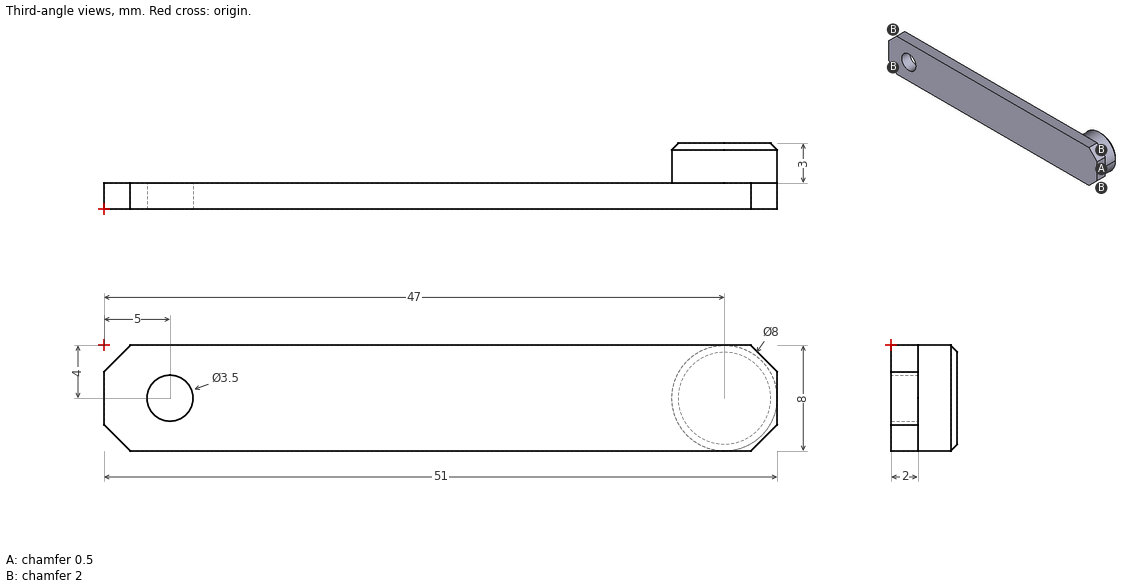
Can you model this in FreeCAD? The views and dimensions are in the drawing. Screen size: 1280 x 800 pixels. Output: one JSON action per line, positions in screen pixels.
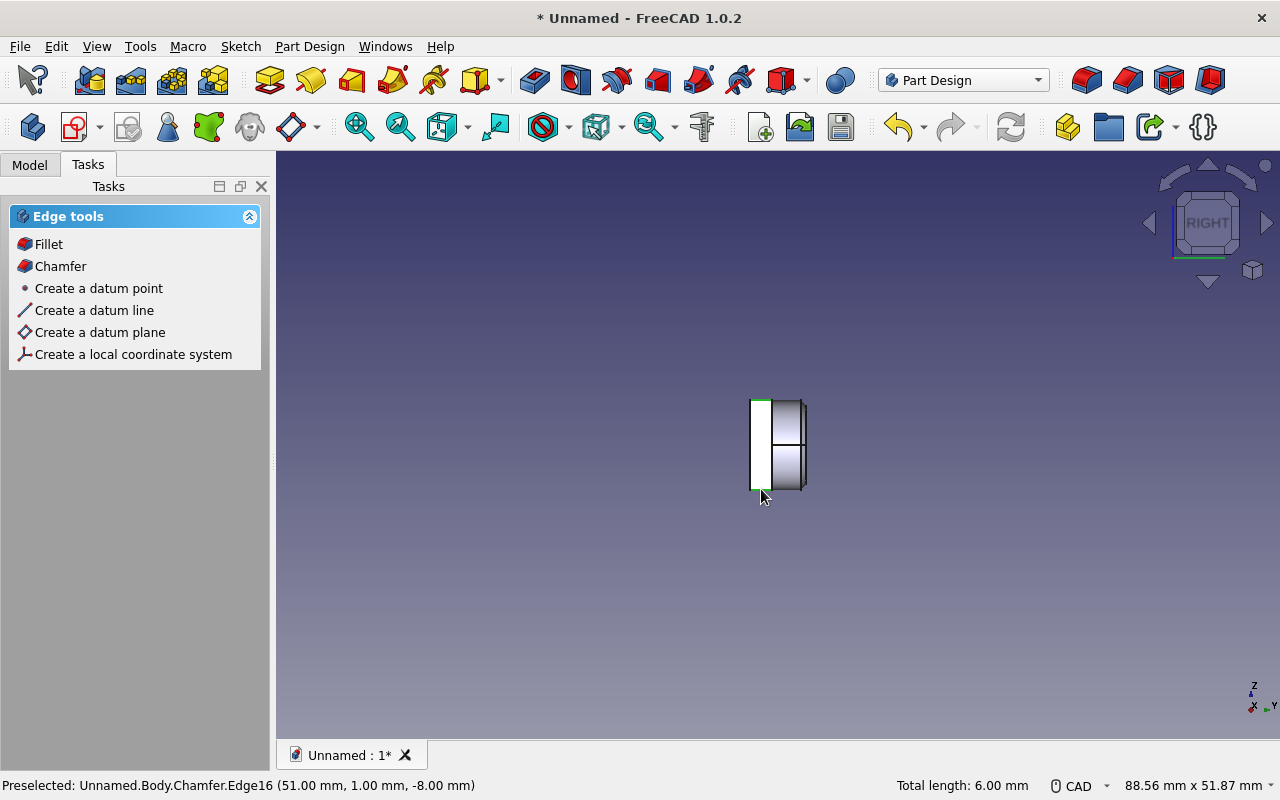
{"action": "key", "text": "5"}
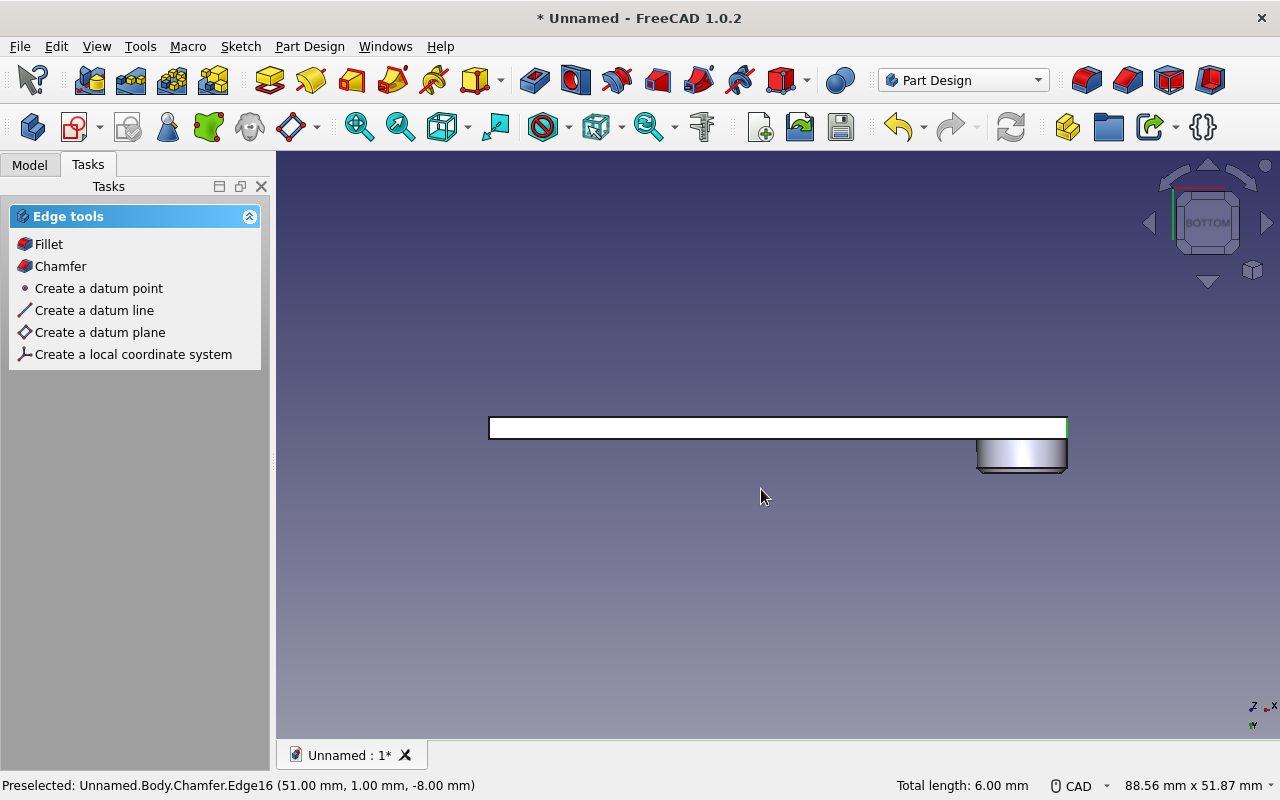
{"action": "left_click", "coordinate": [489, 427], "text": "ctrl"}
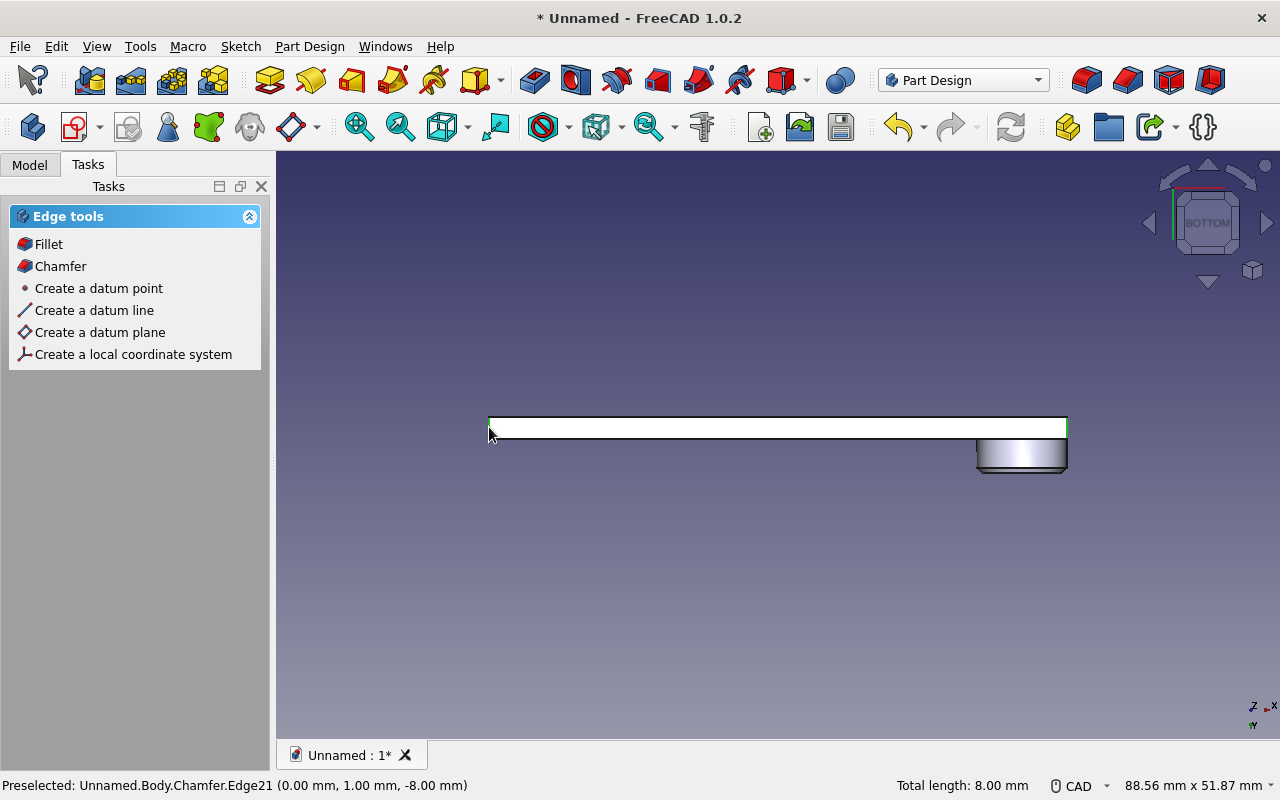
{"action": "left_click", "coordinate": [1128, 80]}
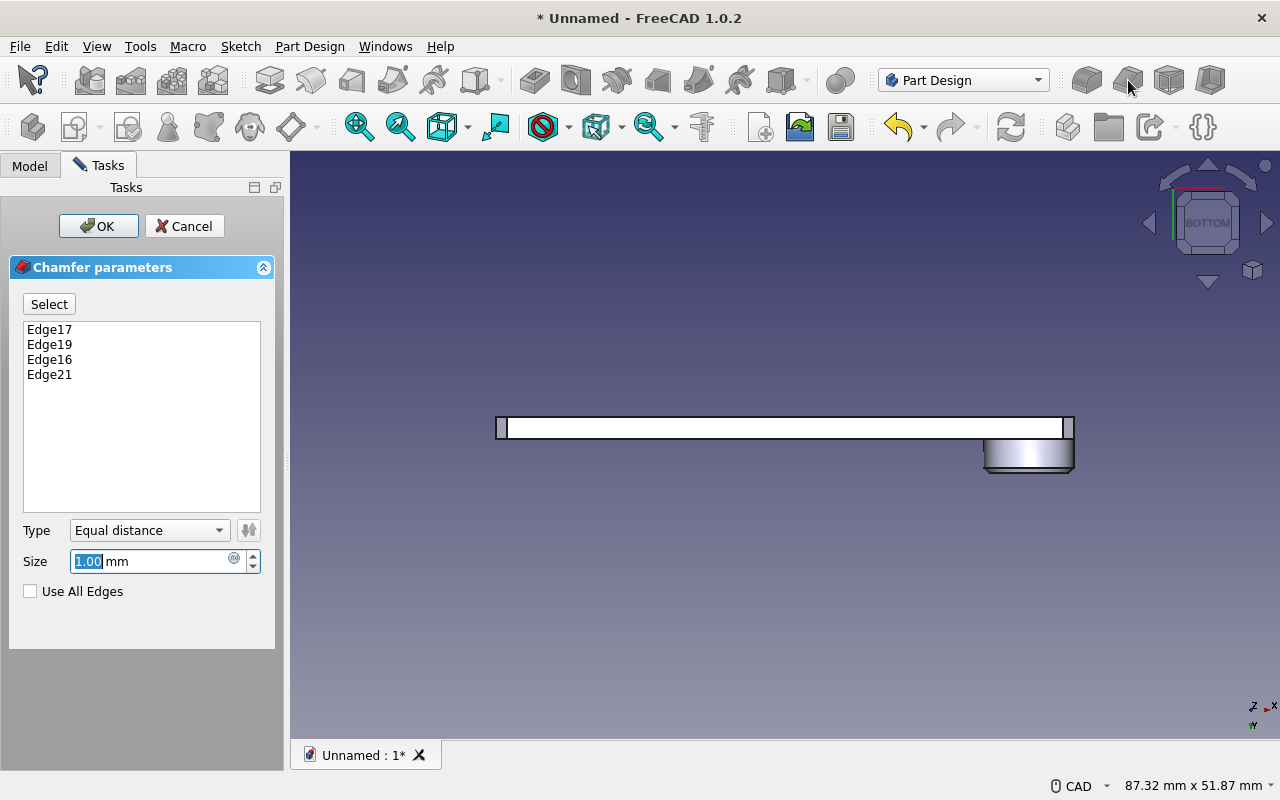
{"action": "type", "text": "2"}
{"action": "key", "text": "Tab"}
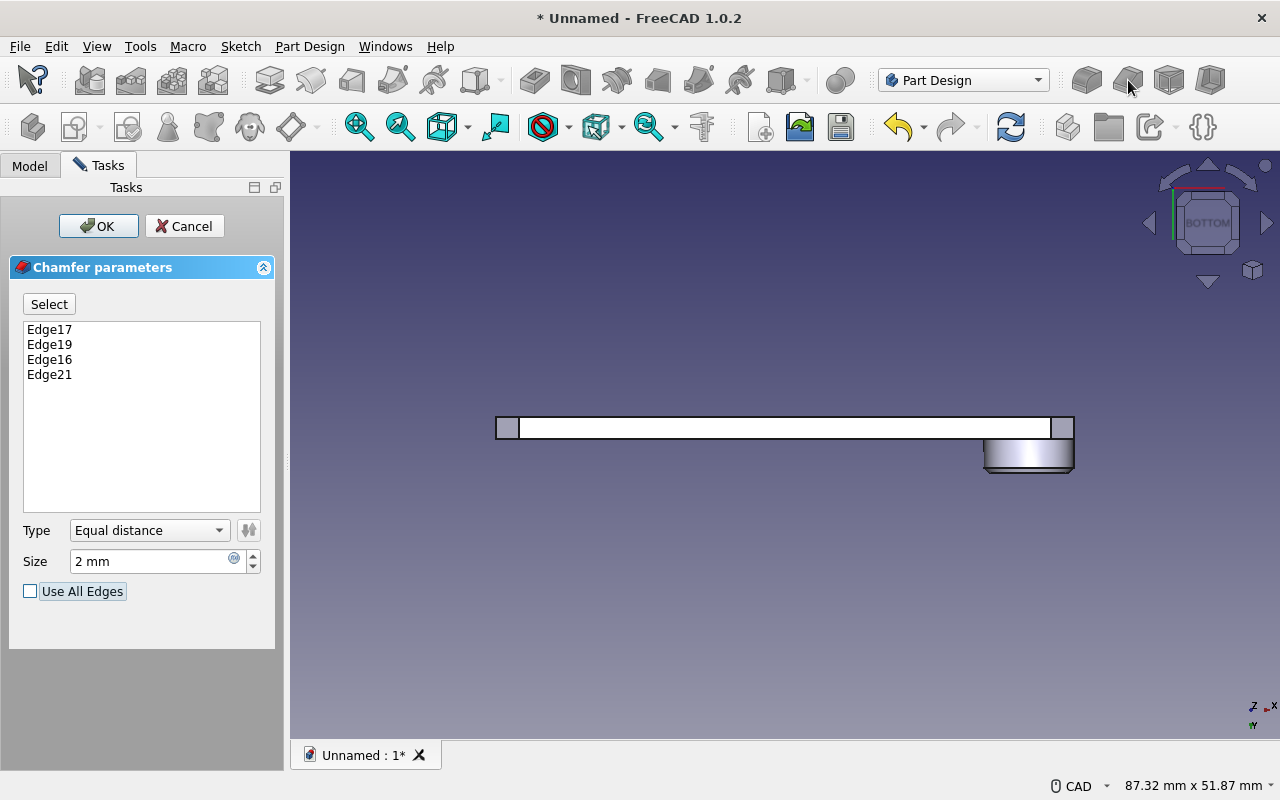
{"action": "left_click", "coordinate": [99, 226]}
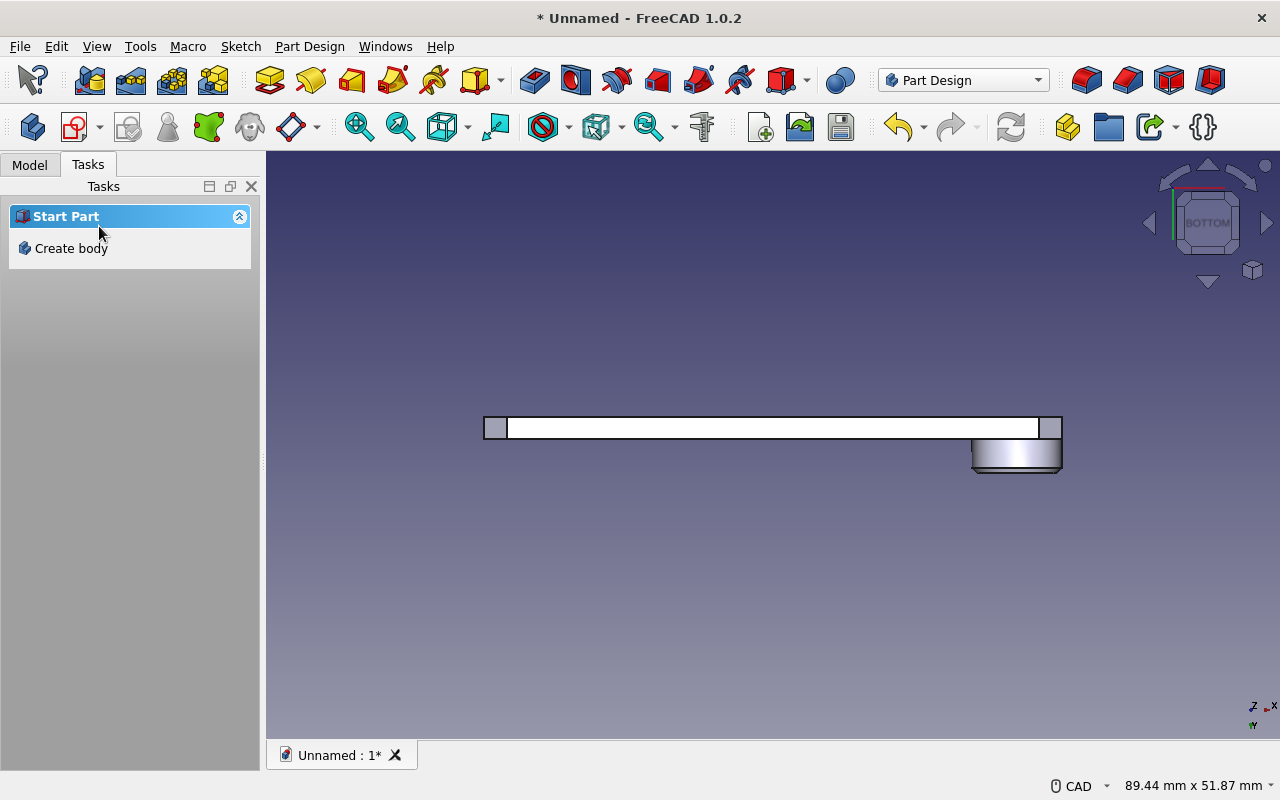
{"action": "key", "text": "0"}